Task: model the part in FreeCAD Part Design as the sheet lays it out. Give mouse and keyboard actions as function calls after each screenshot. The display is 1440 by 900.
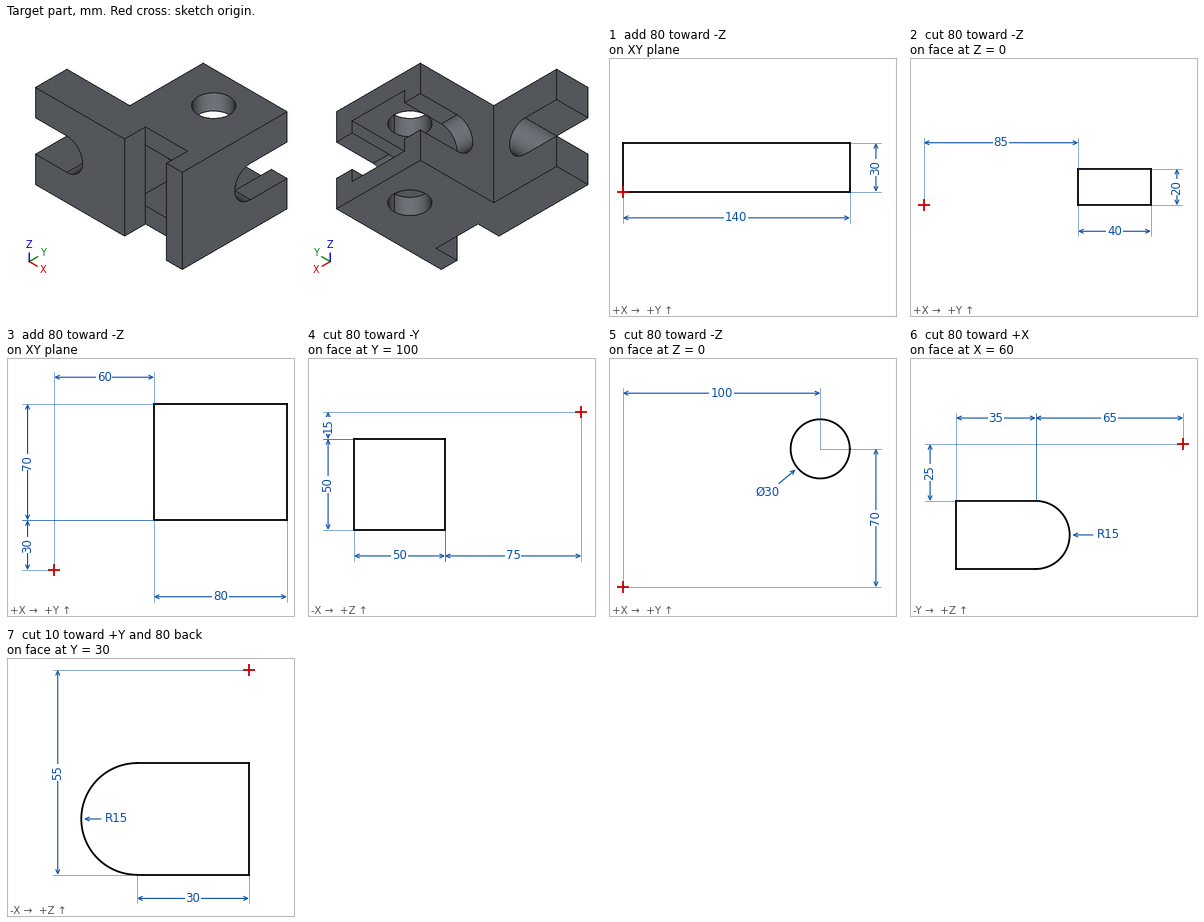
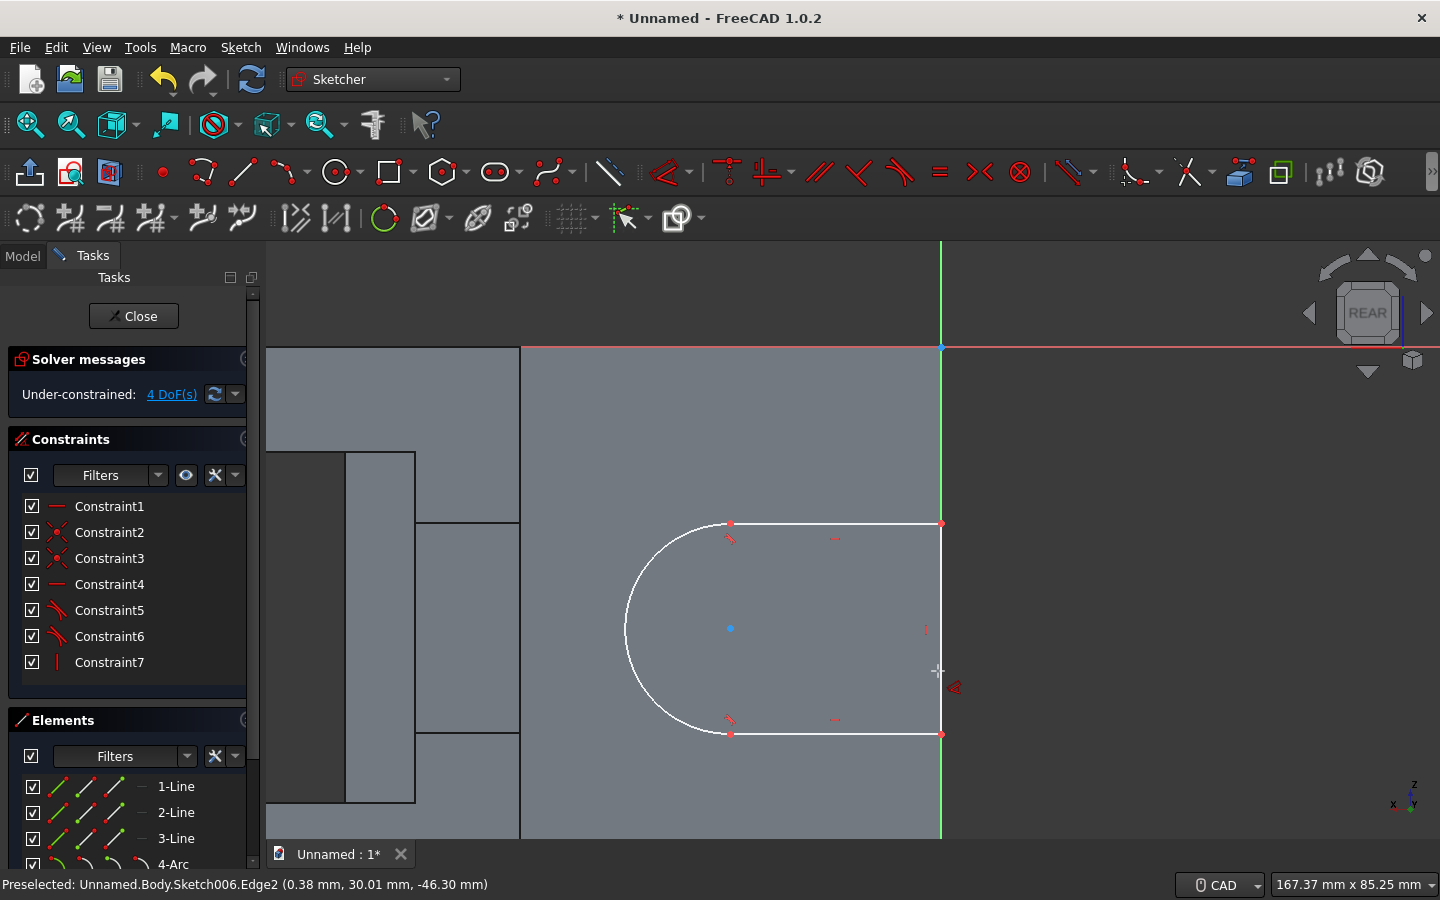
click(645, 567)
click(619, 548)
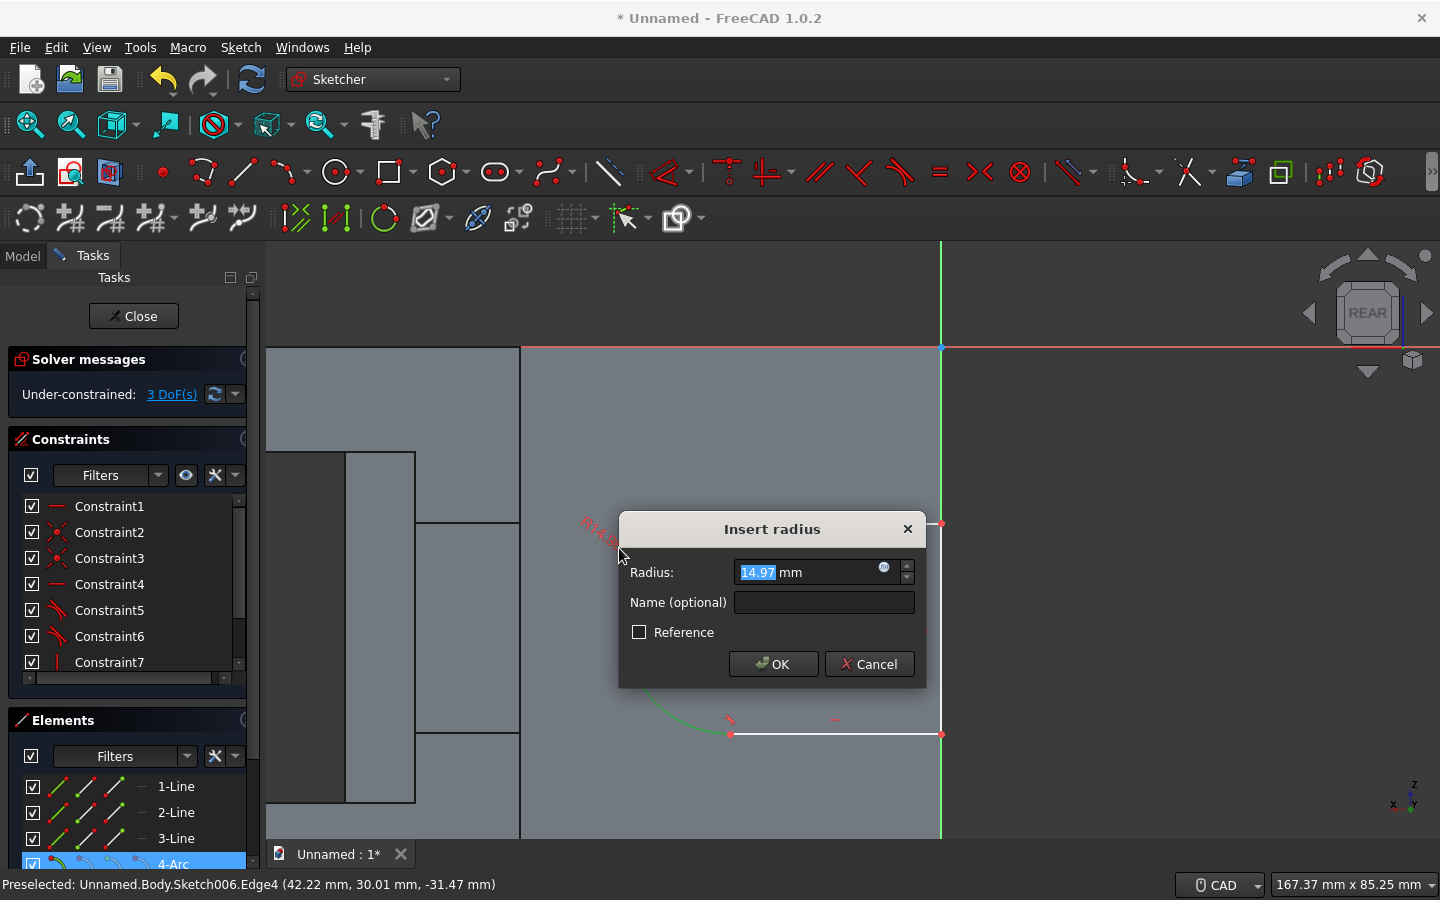
text(15)
key(Return)
key(Escape)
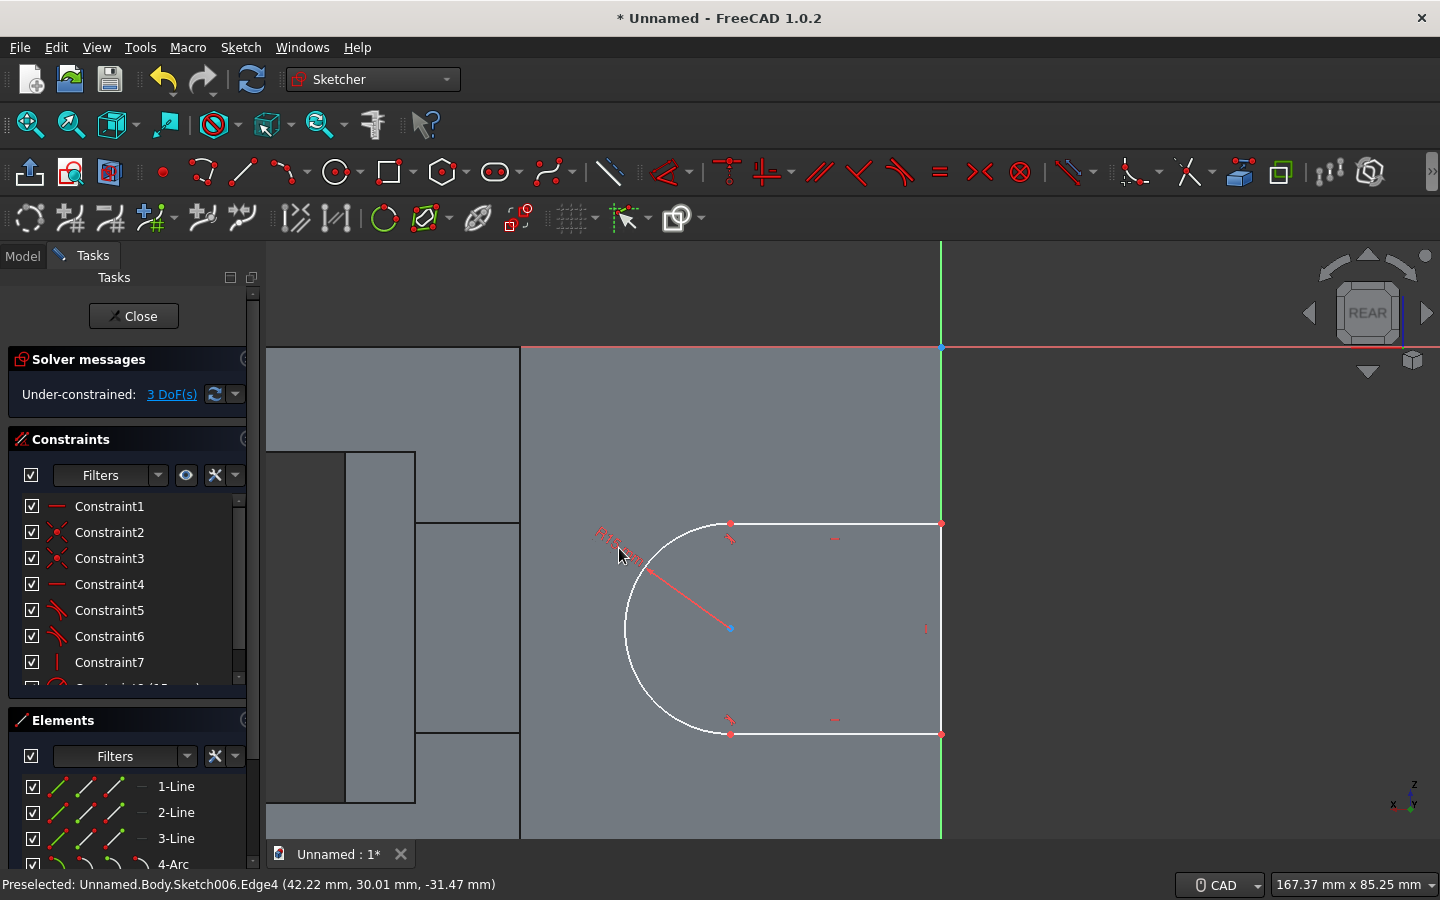
click(941, 734)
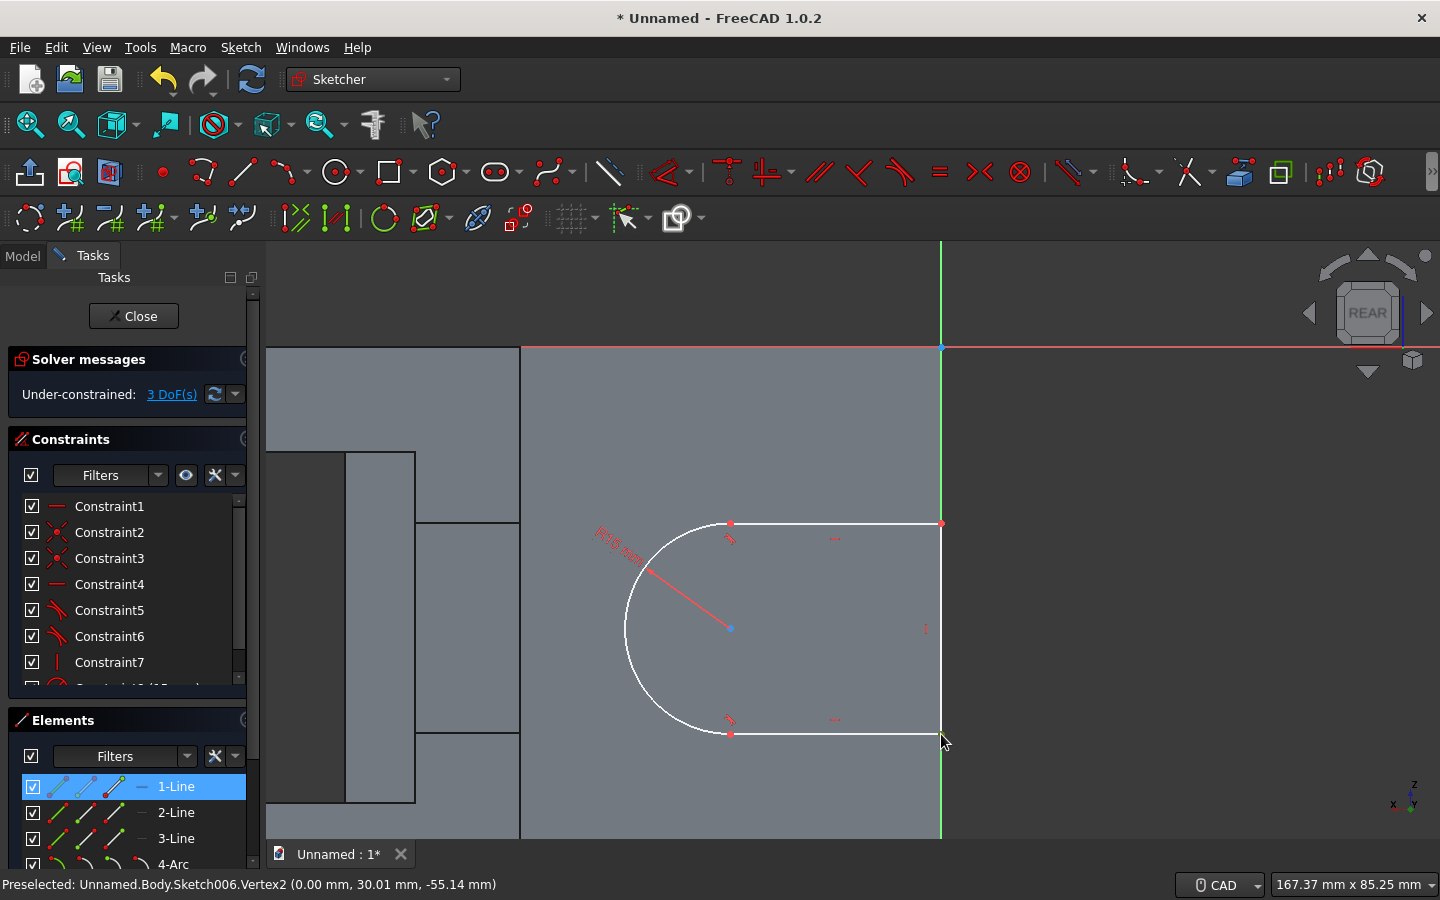
click(941, 772)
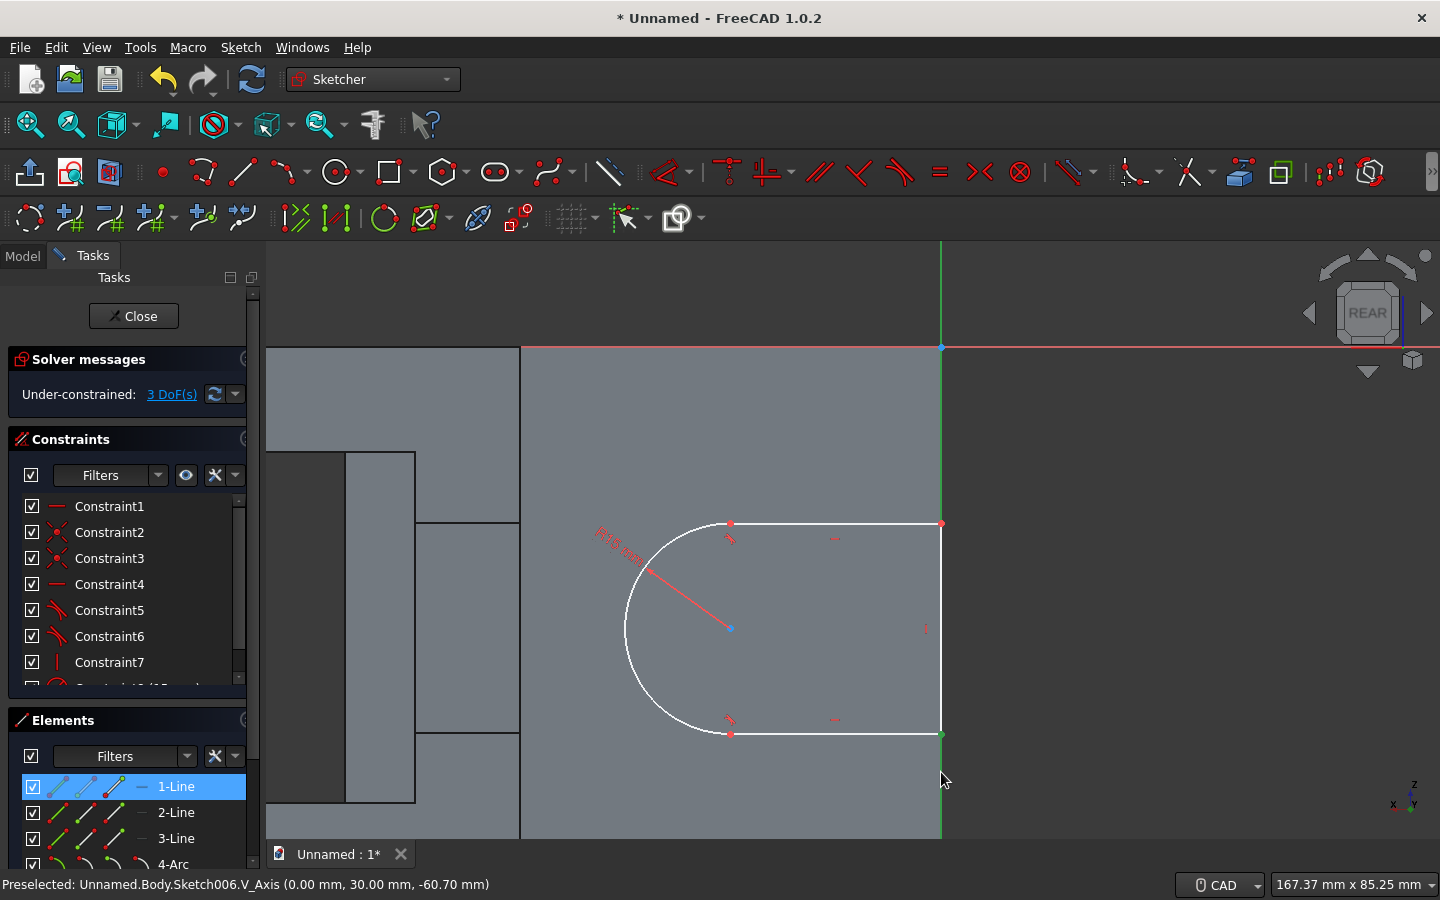
key(c)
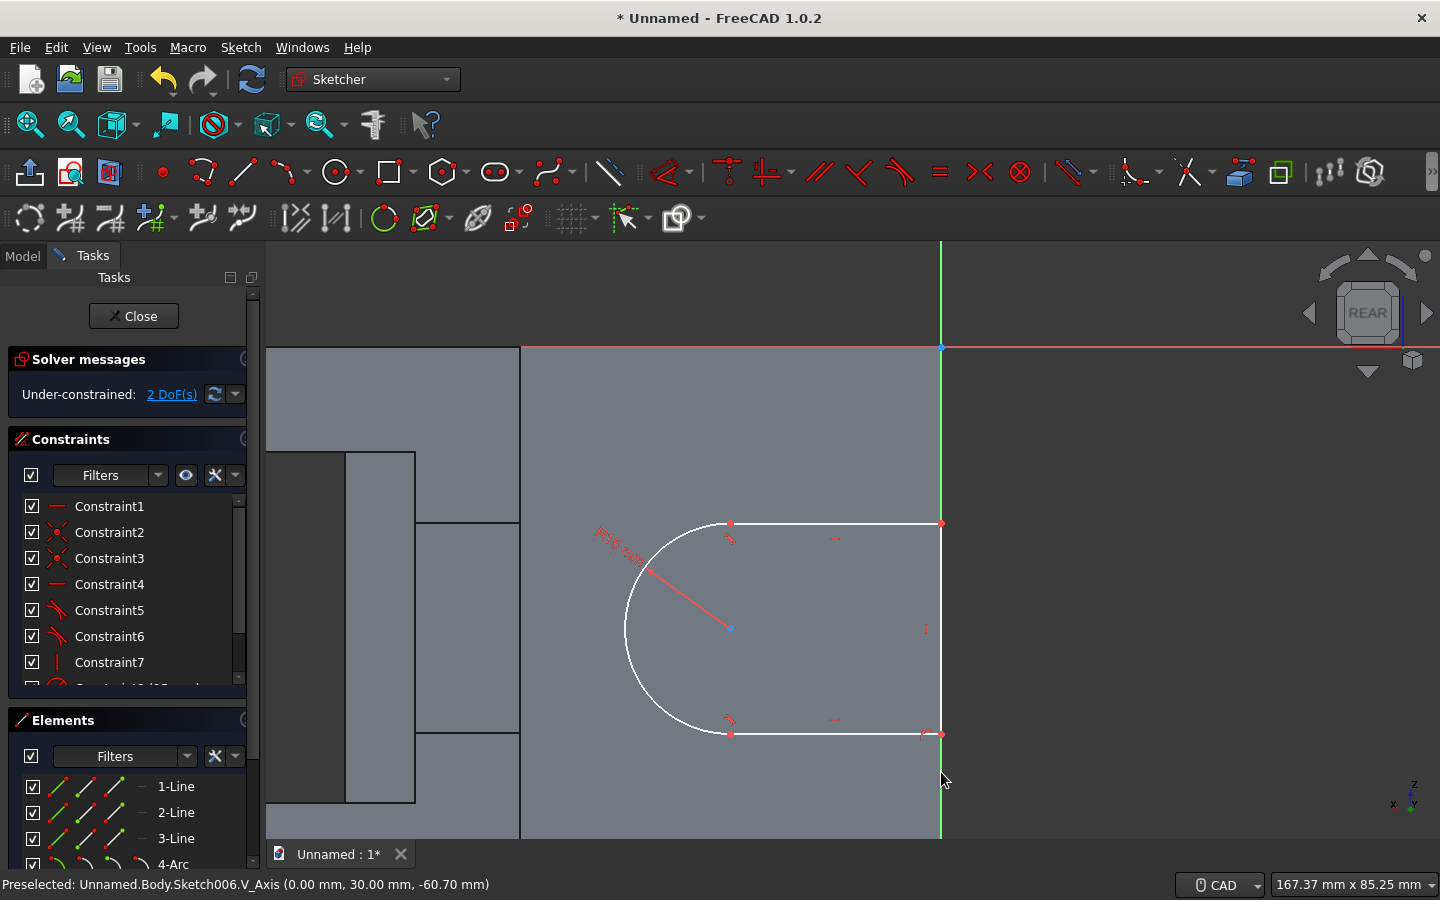
key(d)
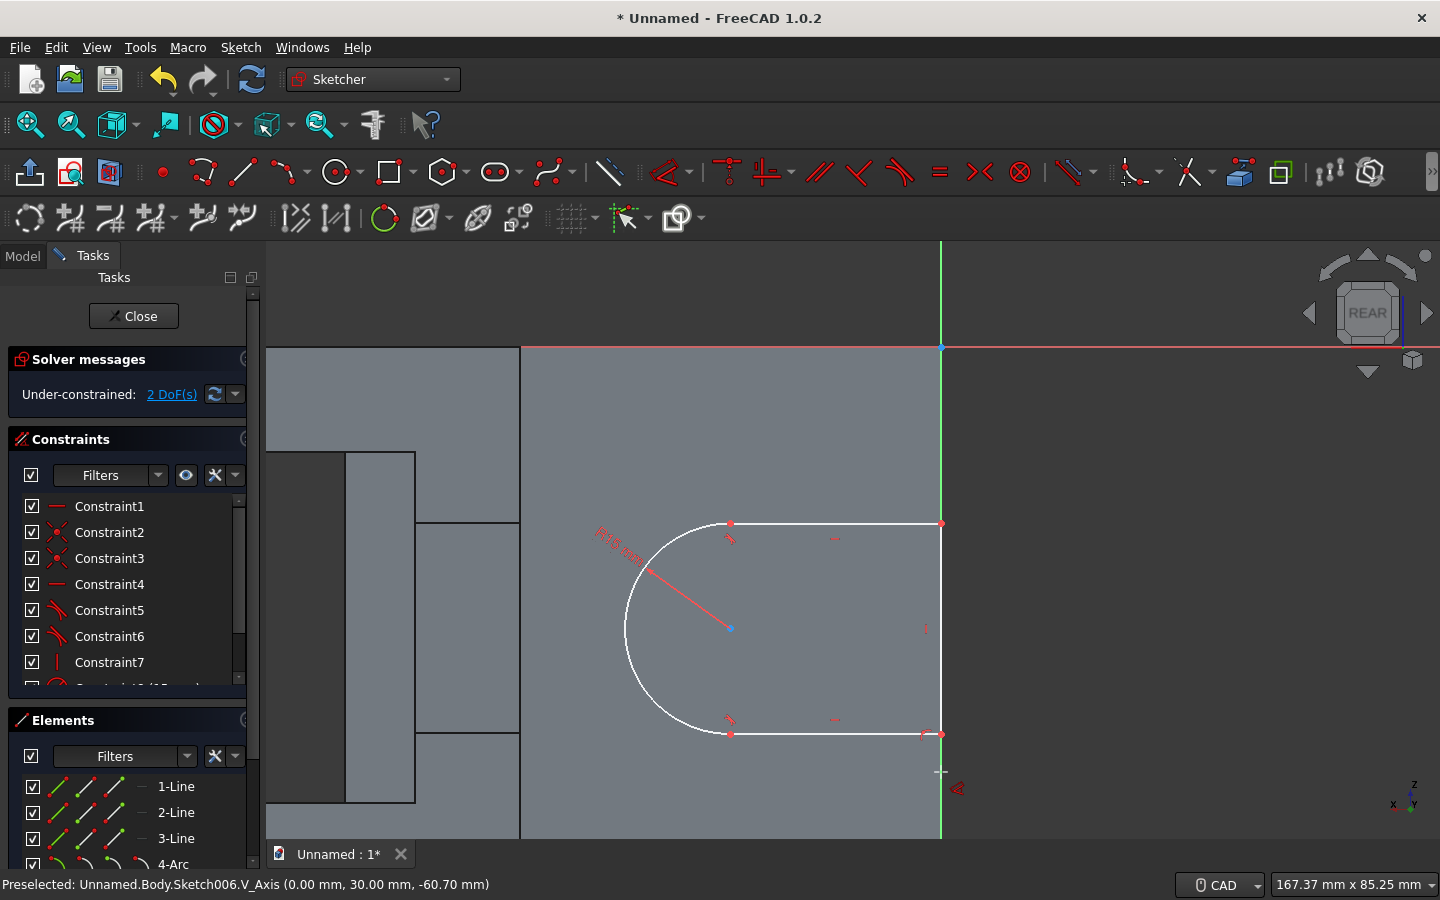
click(794, 734)
click(836, 768)